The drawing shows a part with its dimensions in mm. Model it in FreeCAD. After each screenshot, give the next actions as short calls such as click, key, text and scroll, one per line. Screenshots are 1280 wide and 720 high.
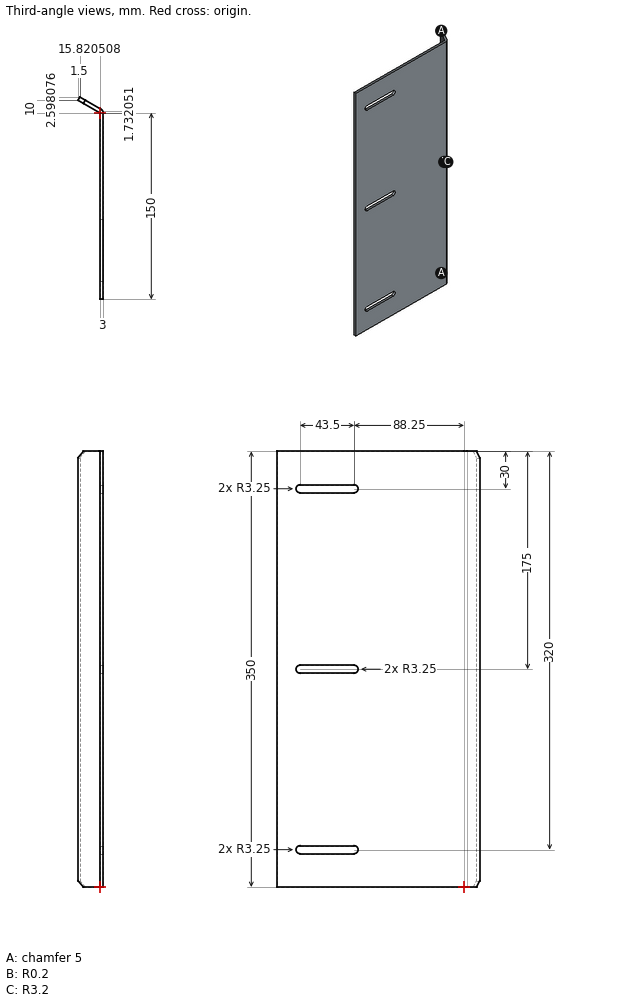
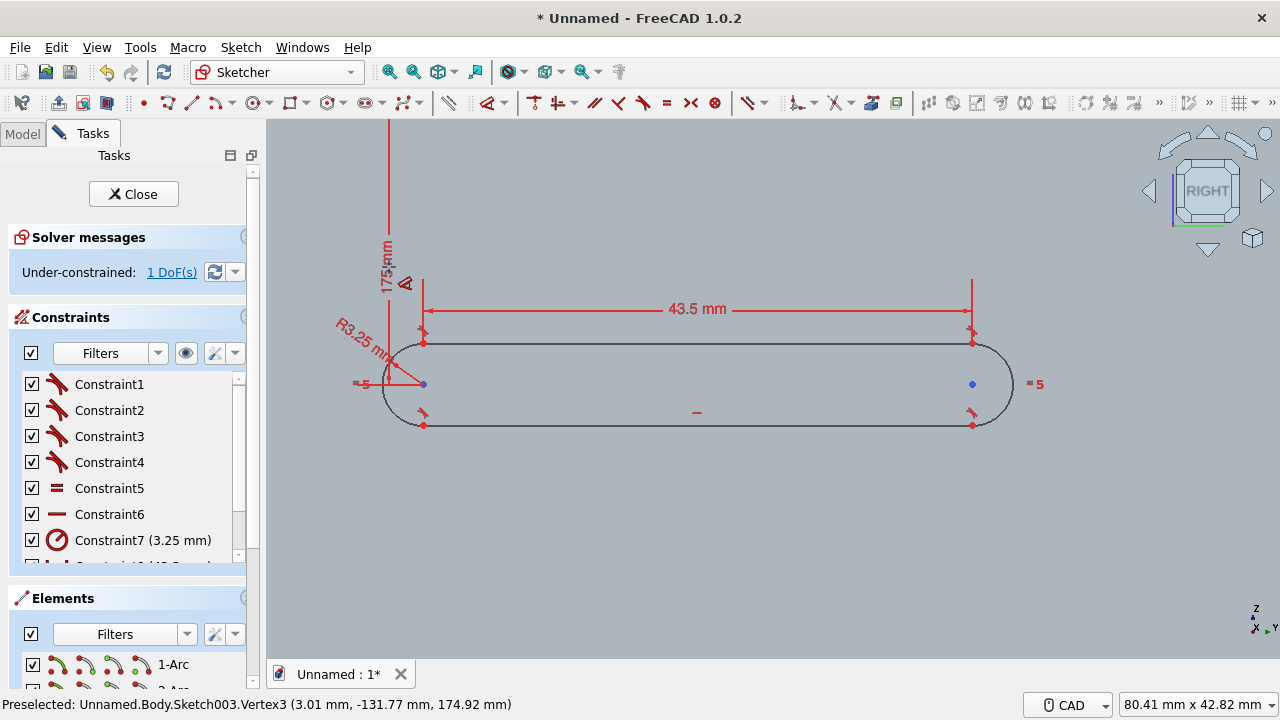
click(972, 426)
click(1044, 460)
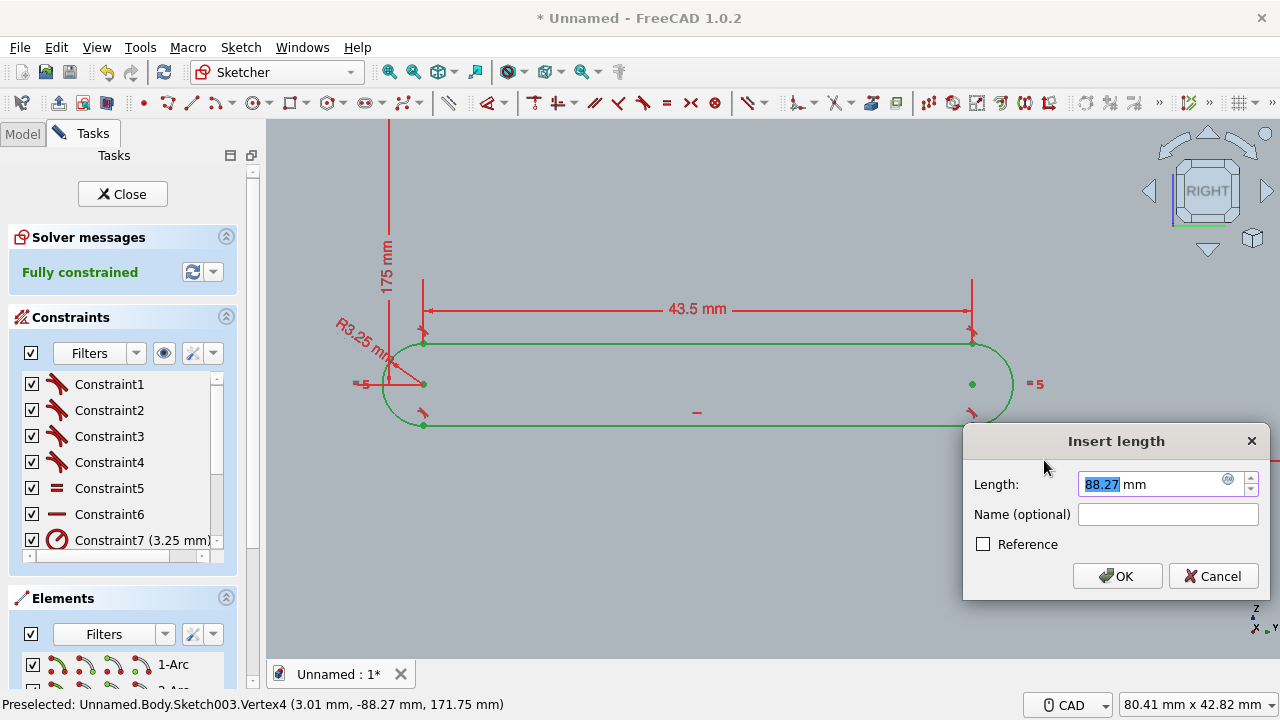
text(88.25)
key(Return)
key(Escape)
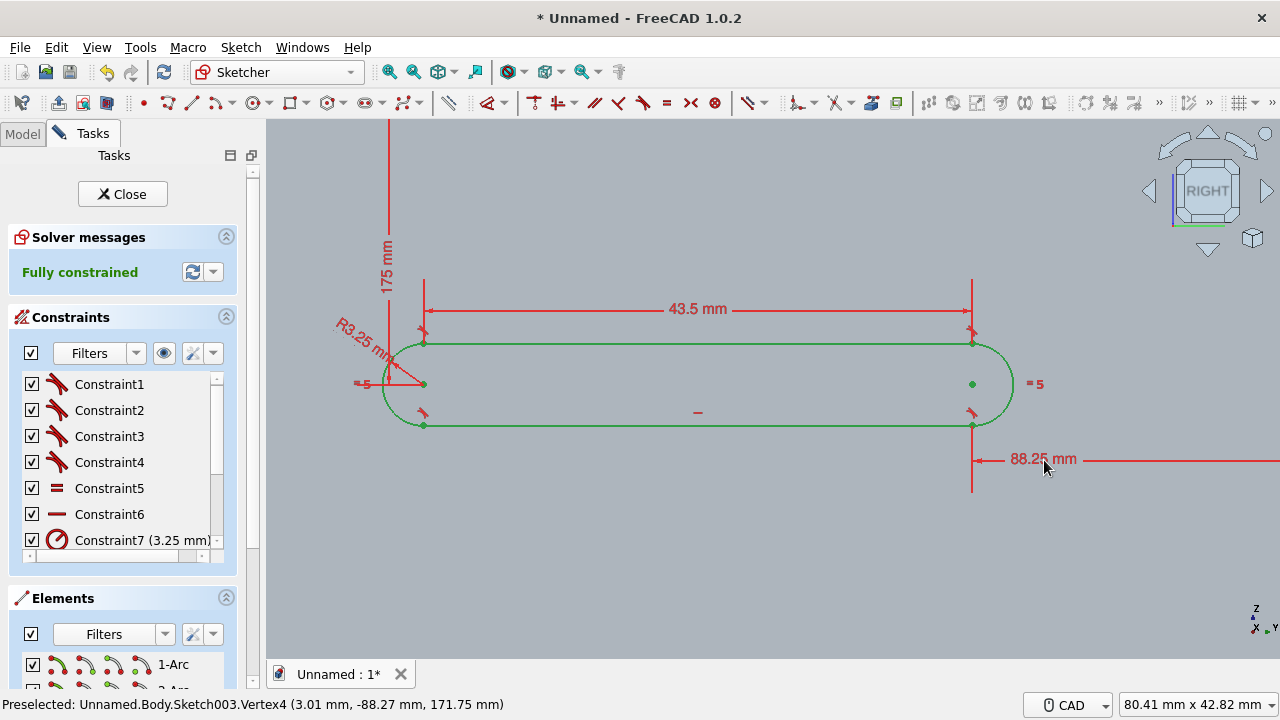
click(123, 194)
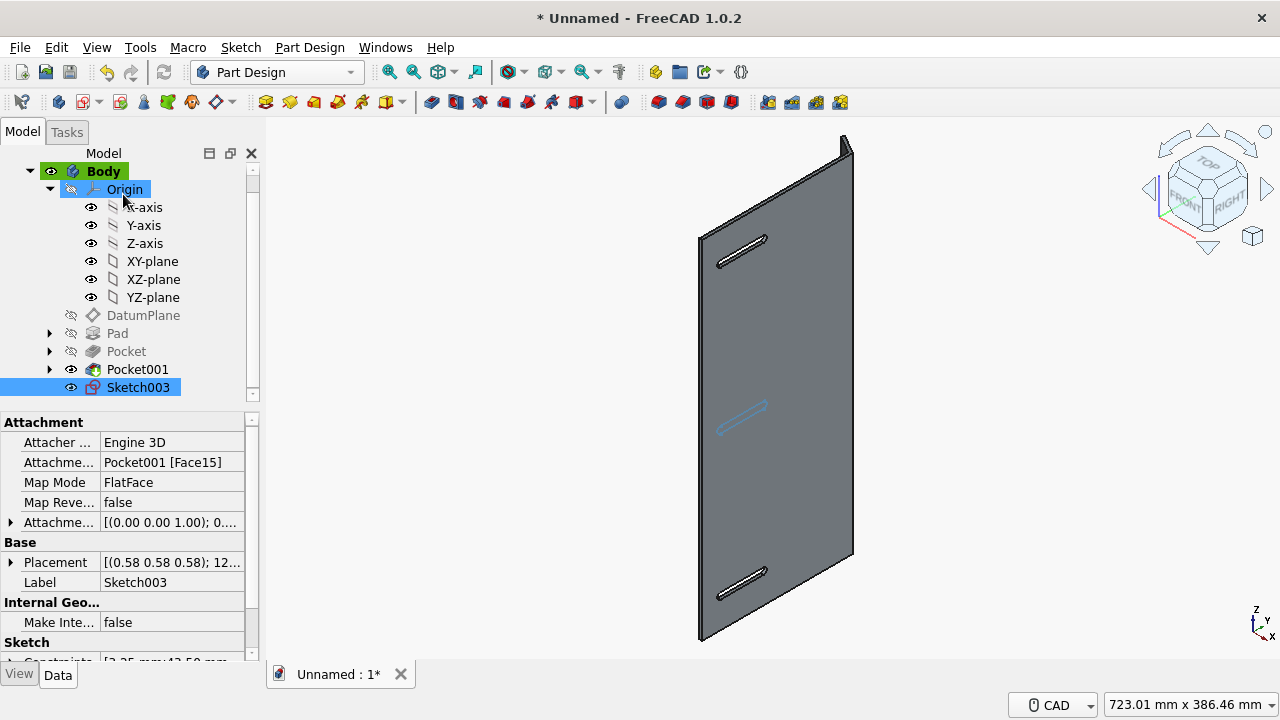
click(432, 102)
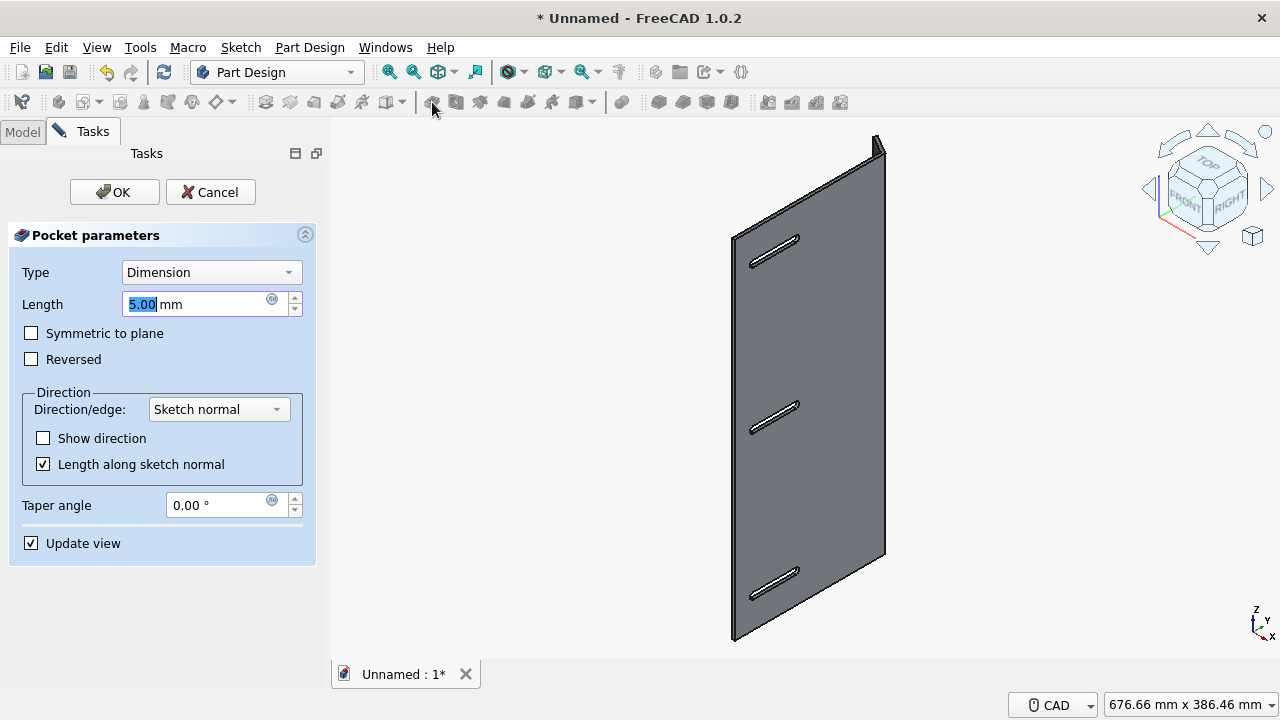
click(212, 272)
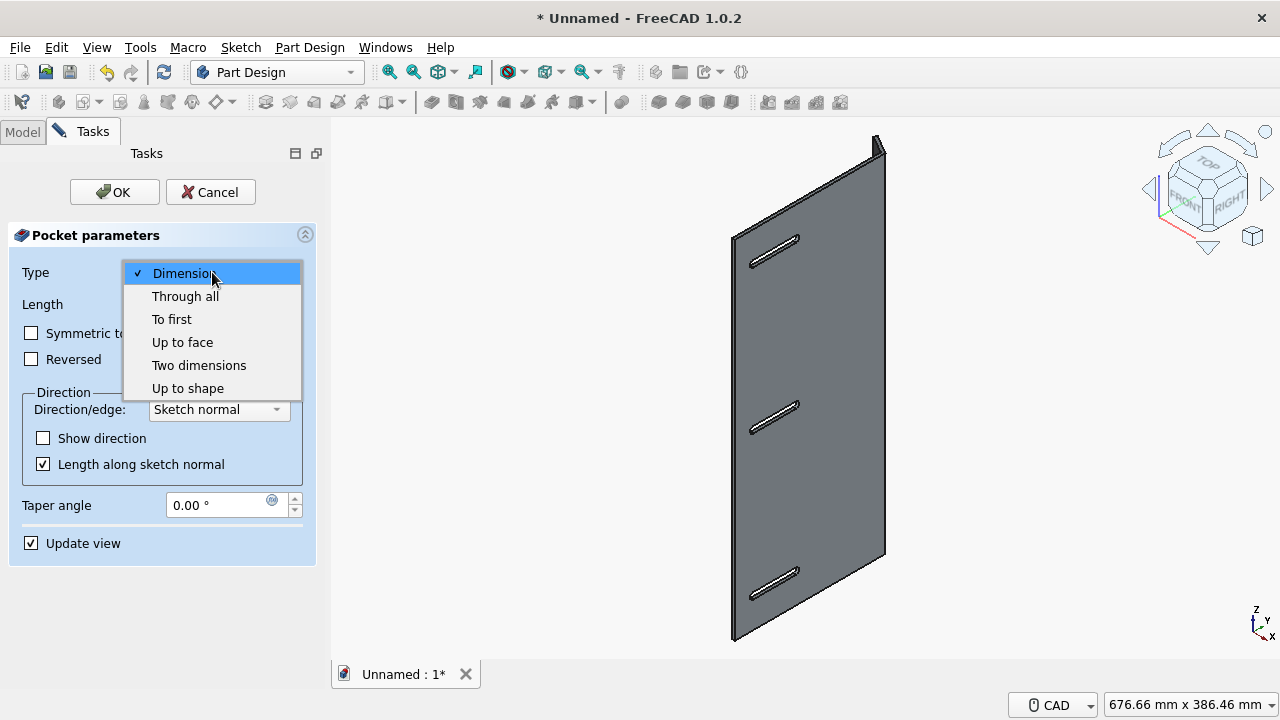
click(212, 296)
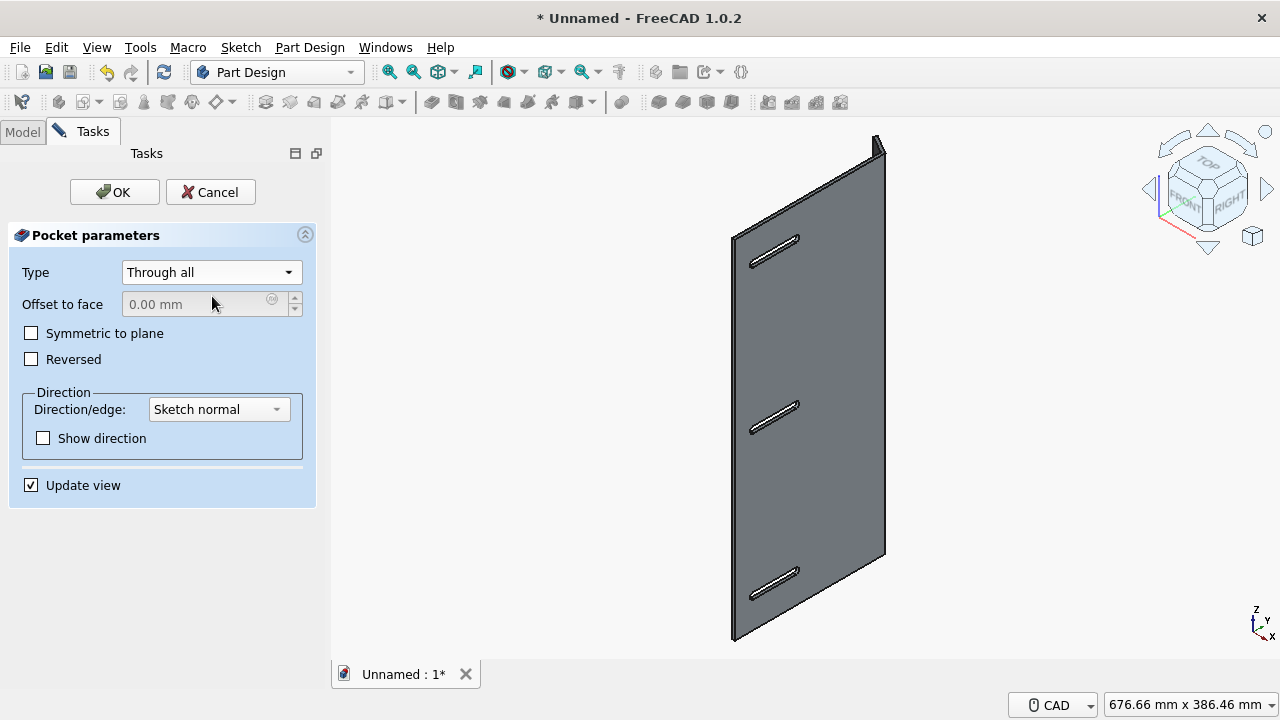
click(115, 192)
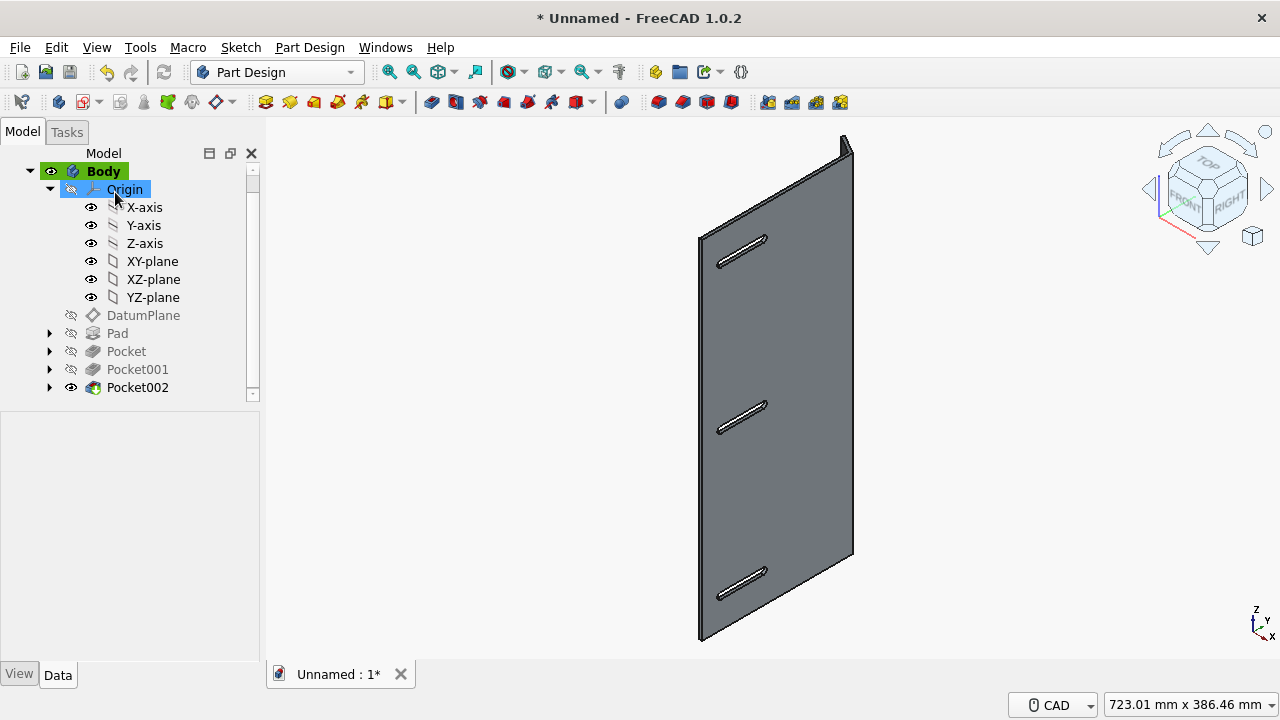
scroll(843, 536, up, 12)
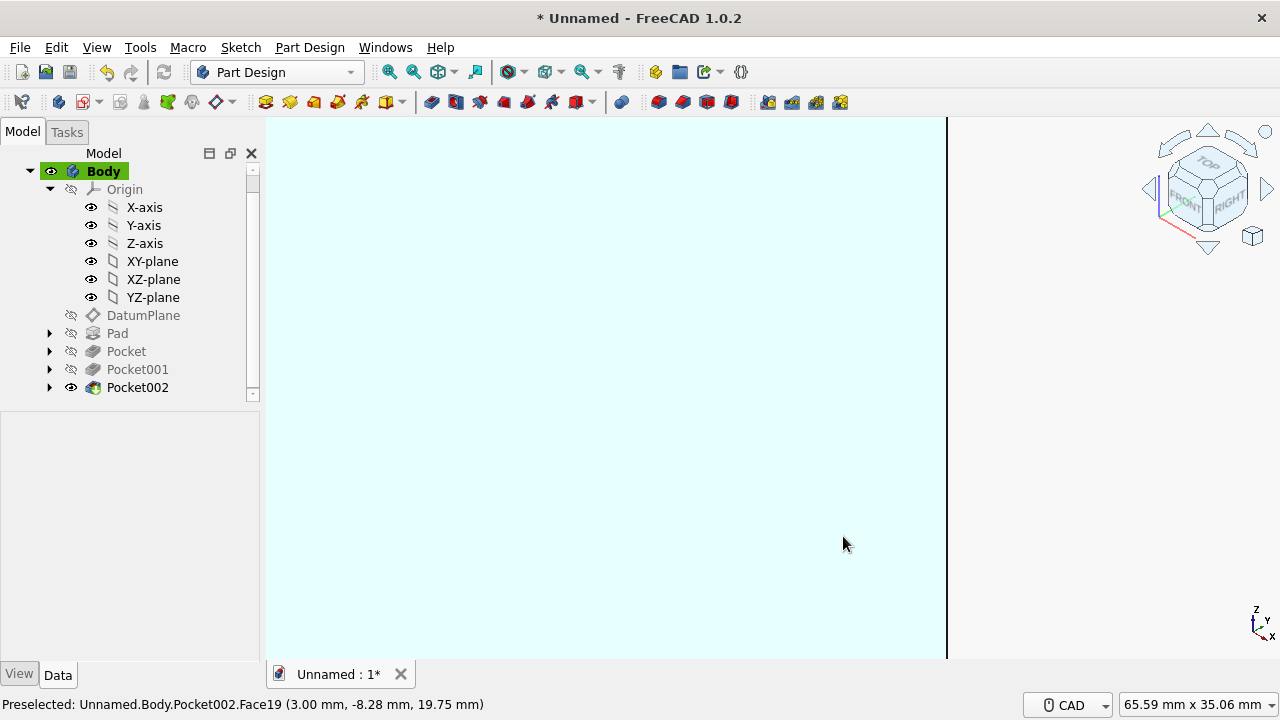
click(390, 72)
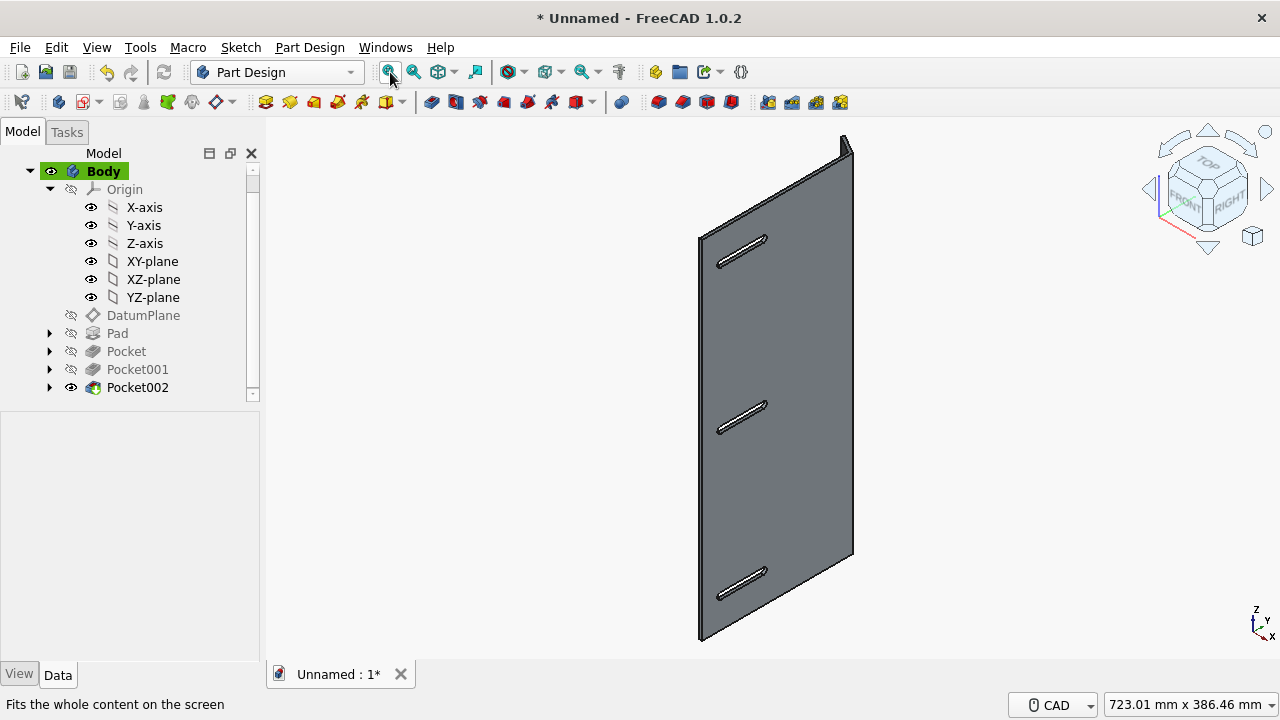
key(2)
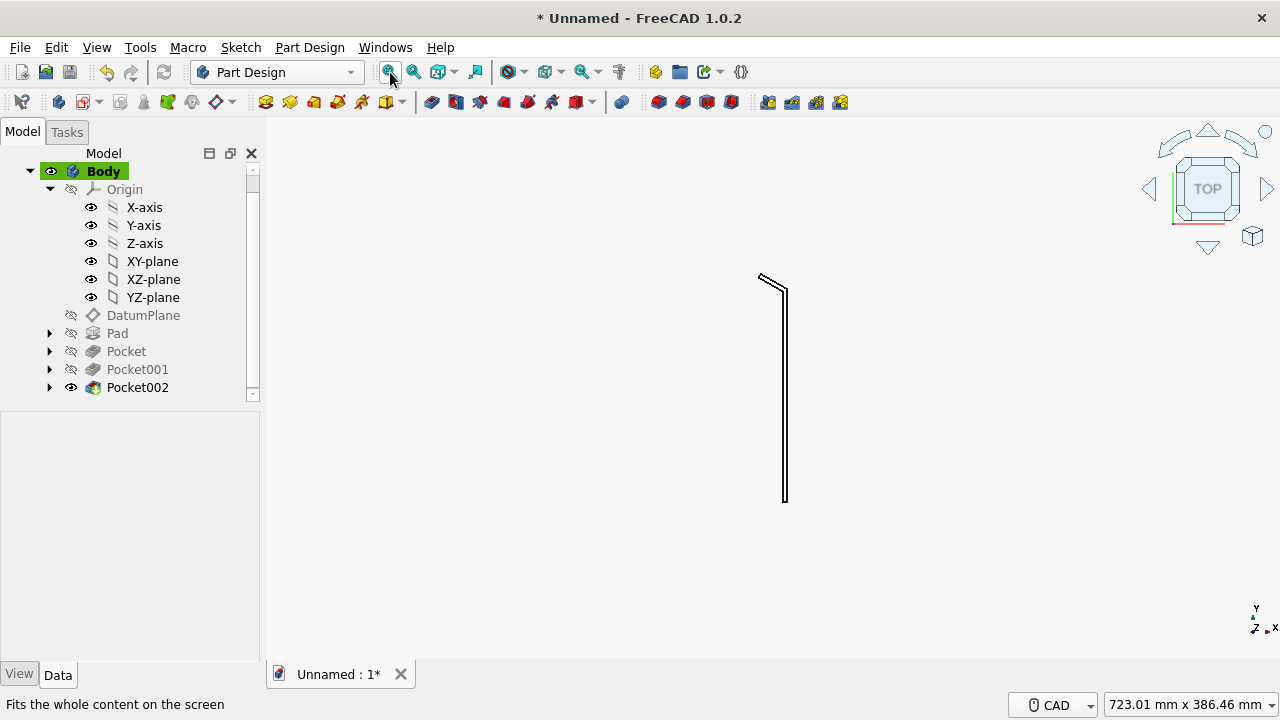
click(390, 72)